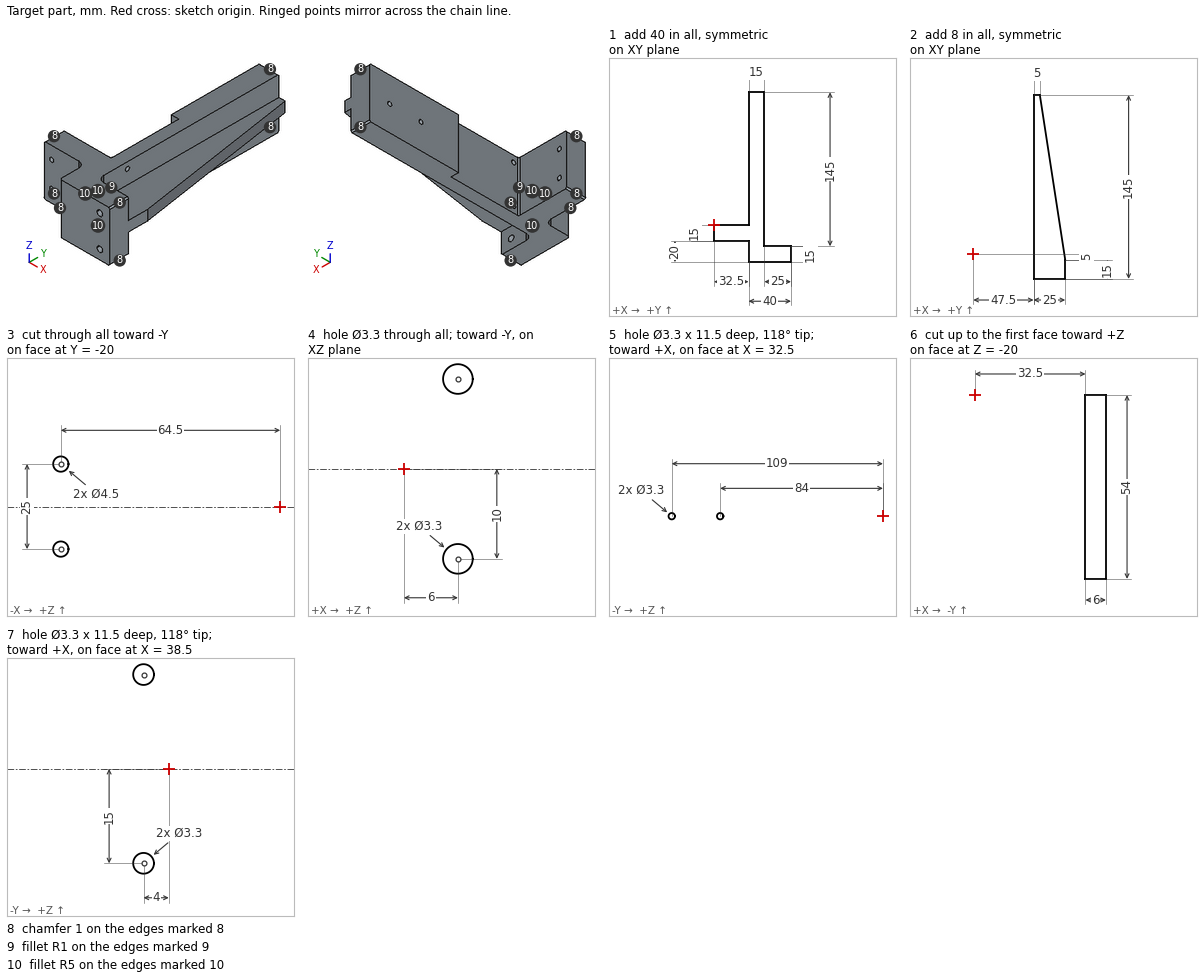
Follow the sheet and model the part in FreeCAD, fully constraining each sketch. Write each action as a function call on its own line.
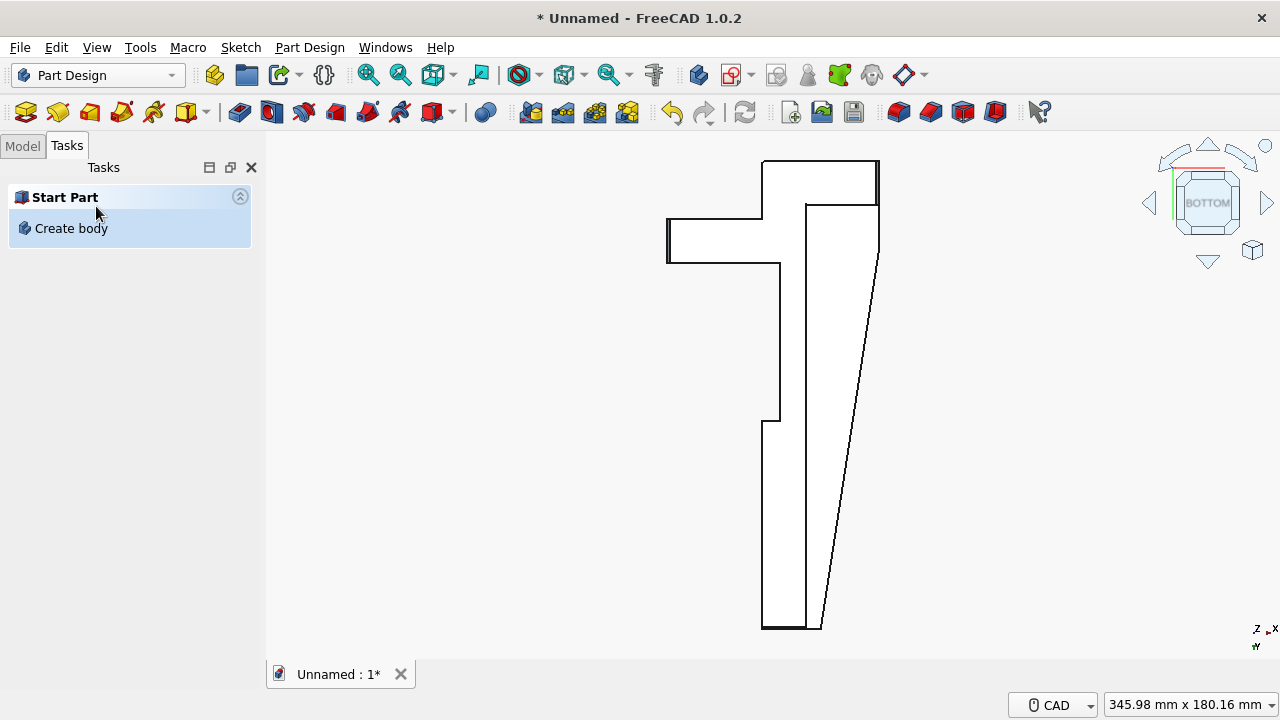
key(0)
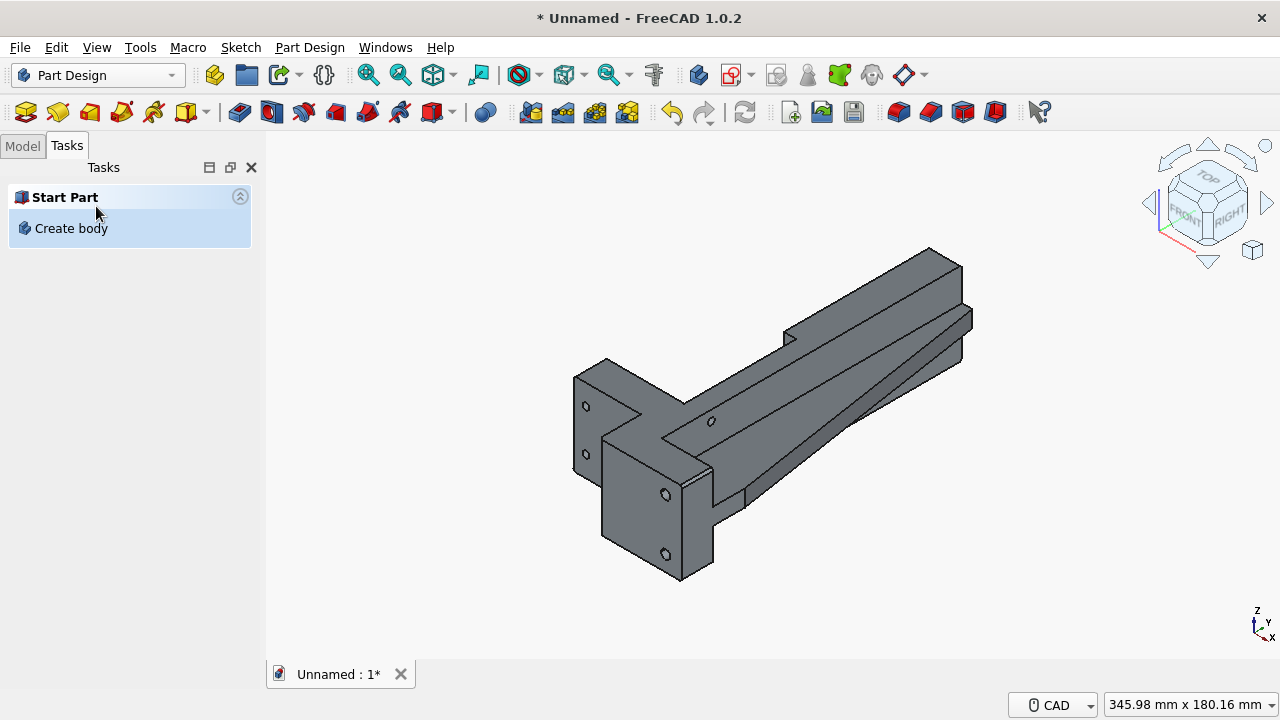
key(2)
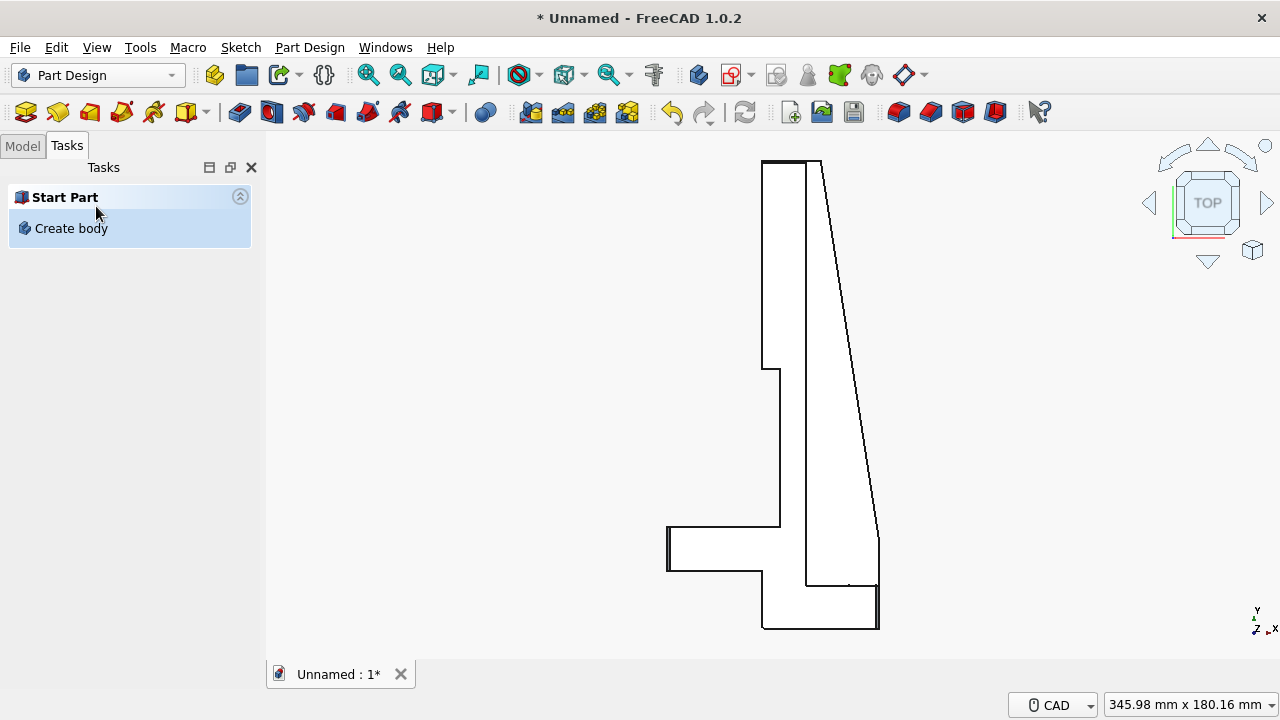
key(1)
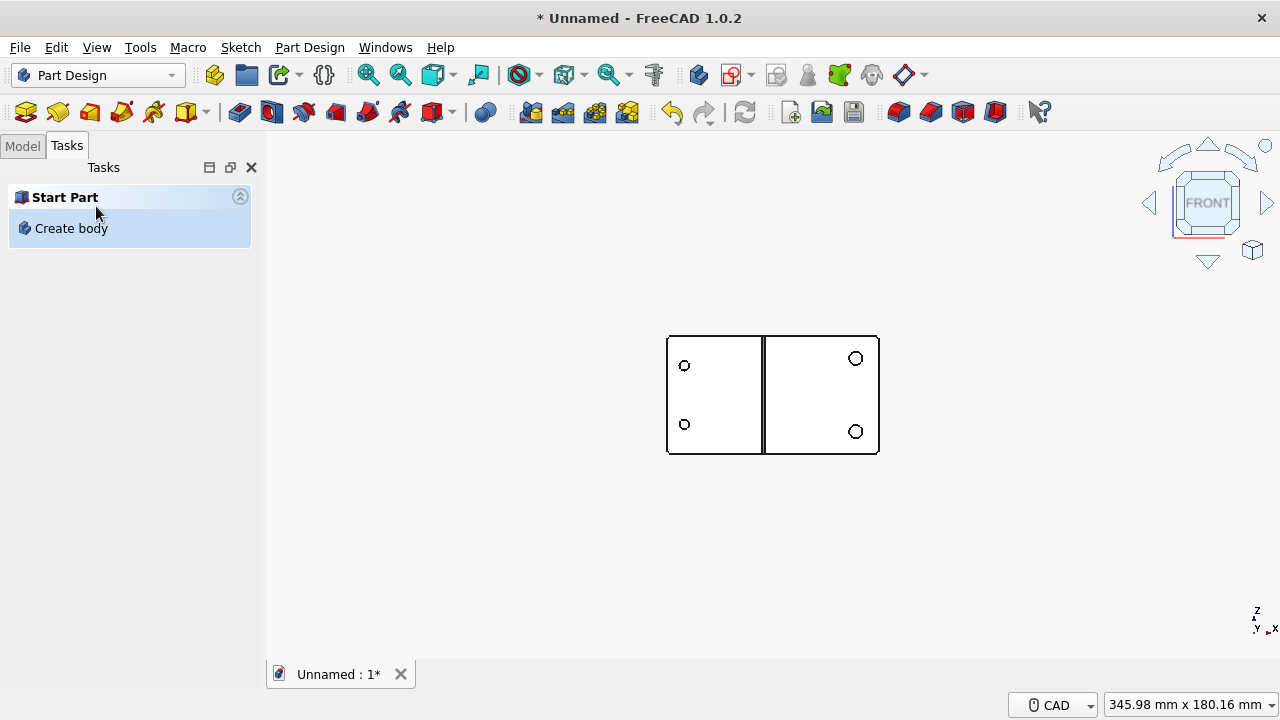
click(370, 76)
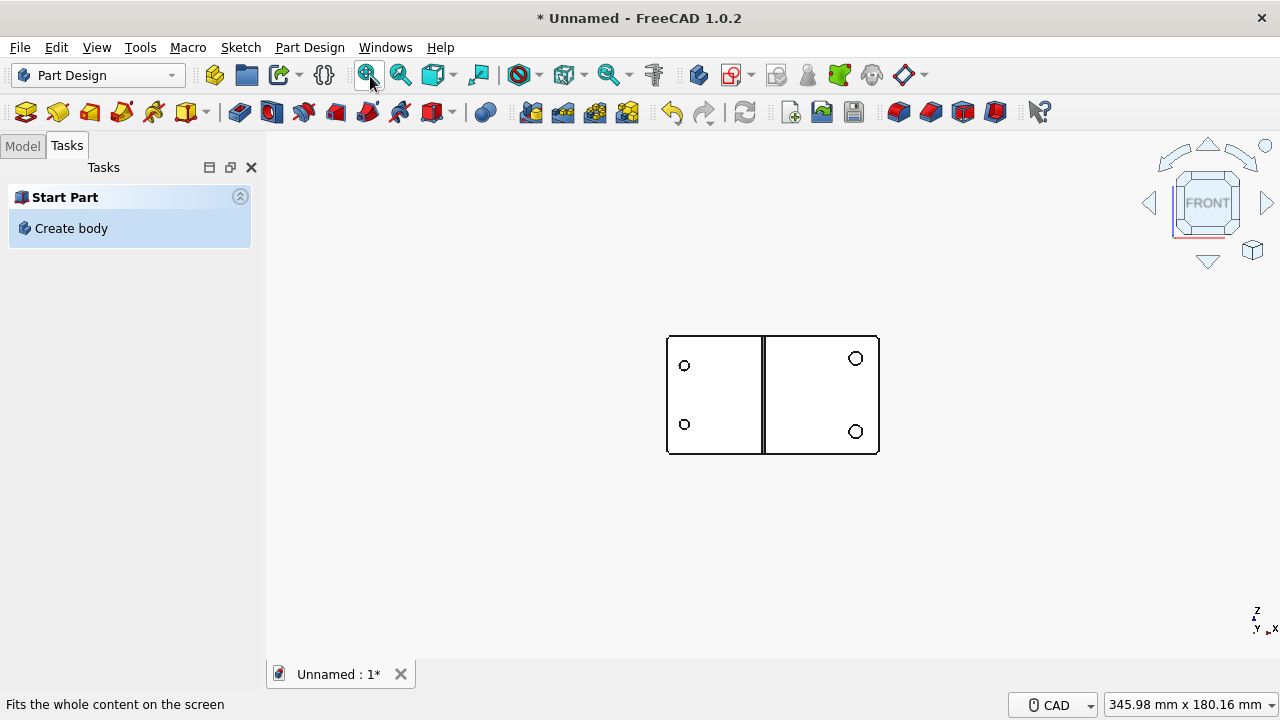
key(3)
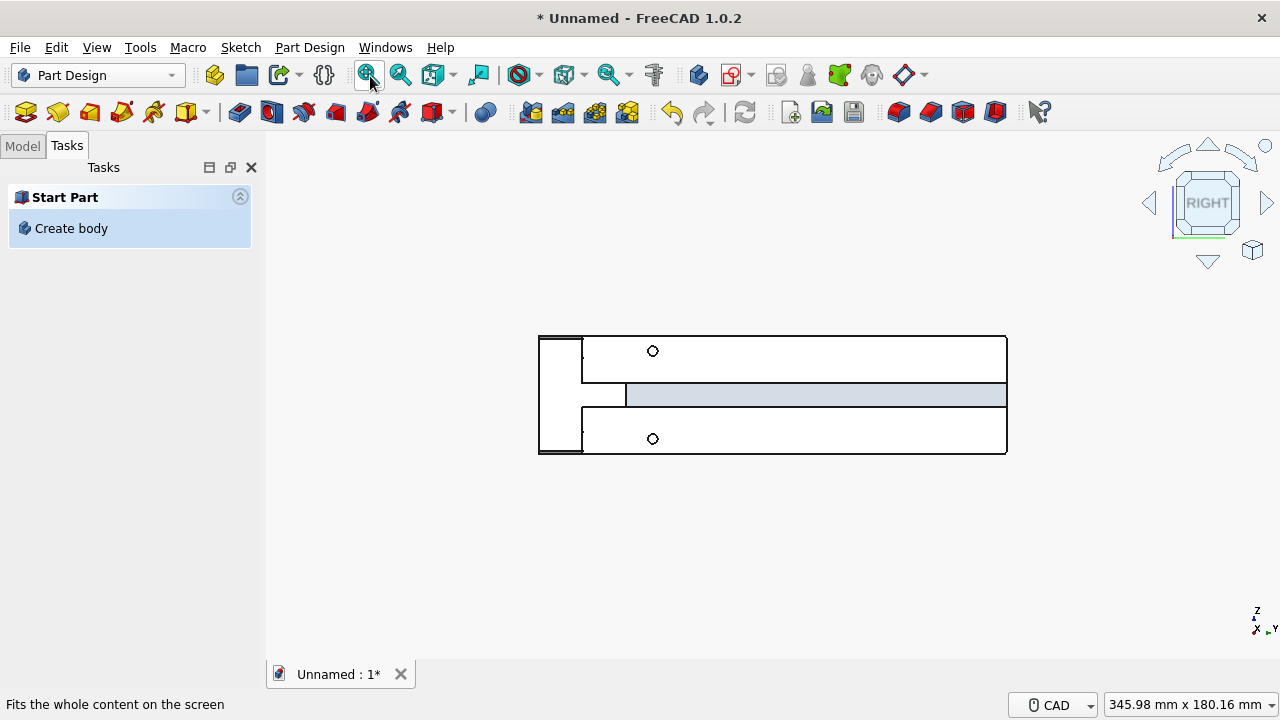
key(5)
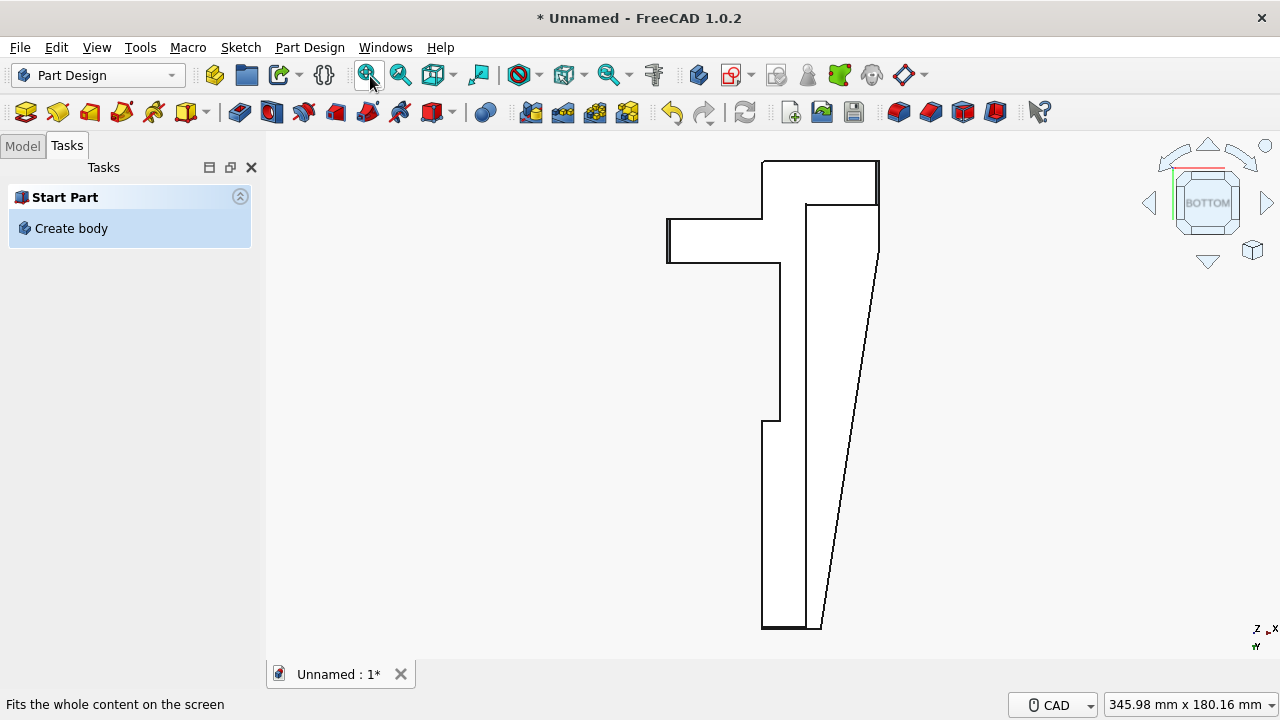
key(4)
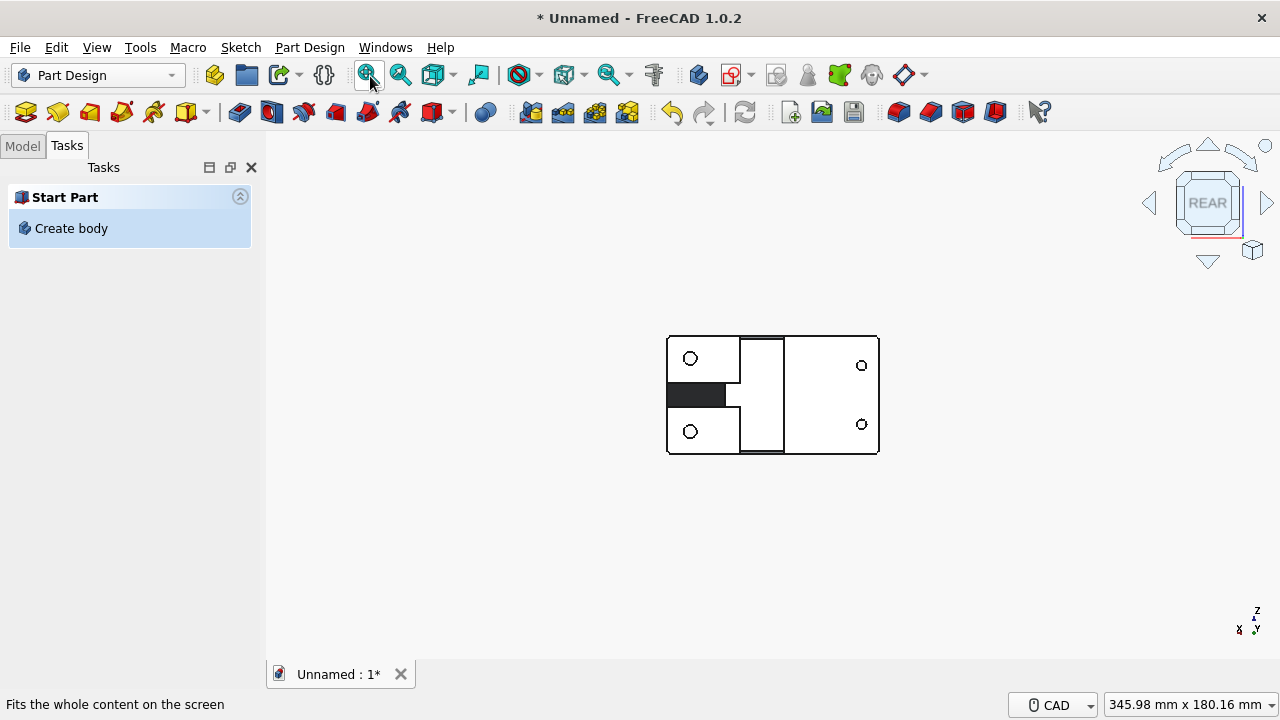
click(370, 76)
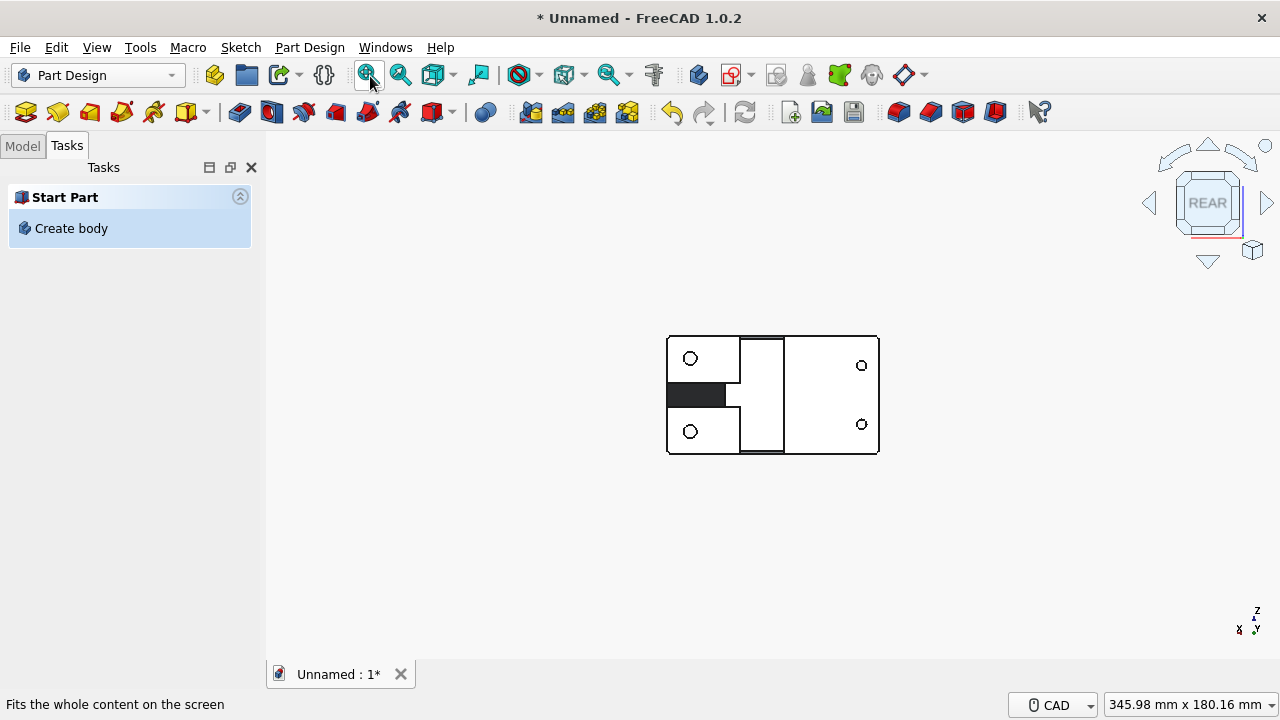
key(6)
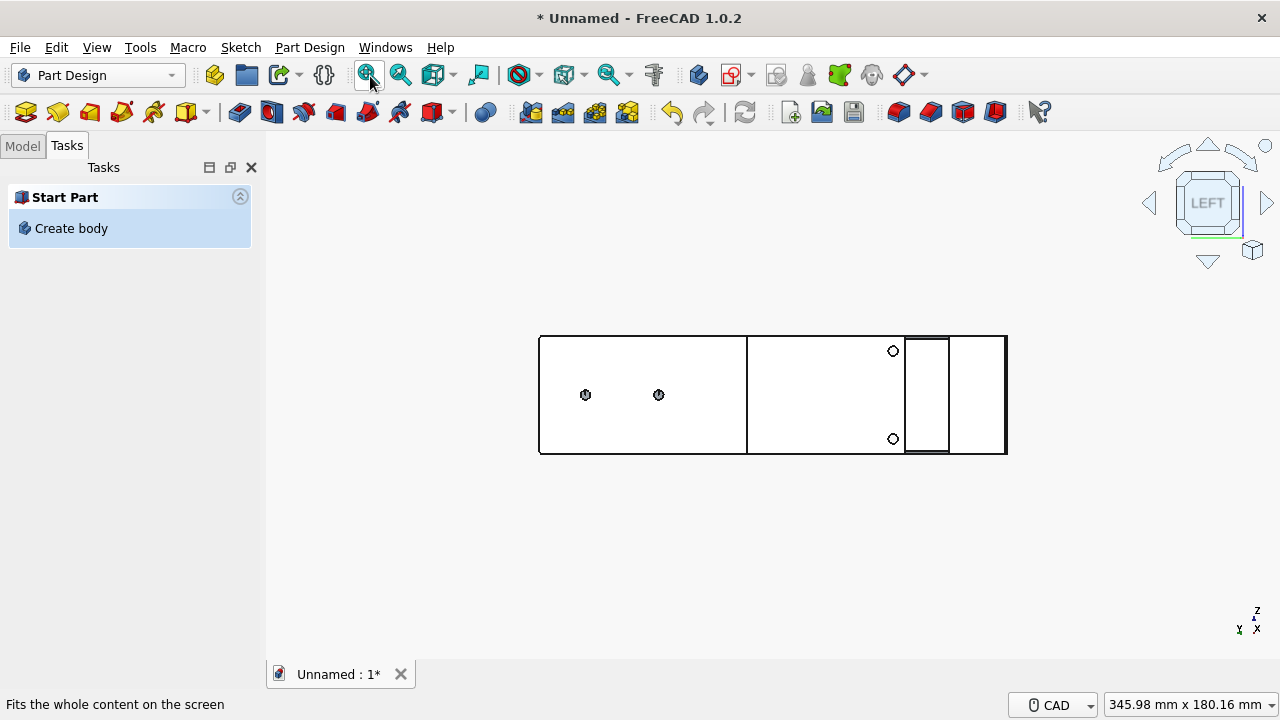
key(v)
key(3)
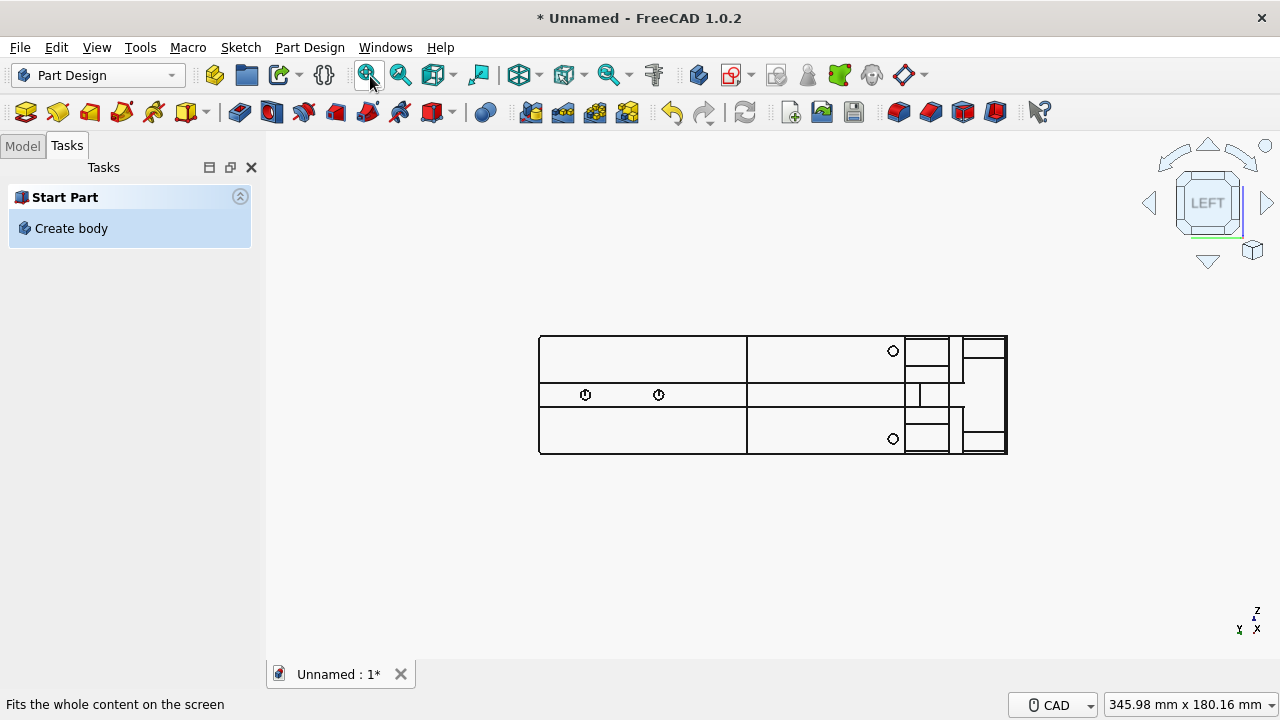
key(0)